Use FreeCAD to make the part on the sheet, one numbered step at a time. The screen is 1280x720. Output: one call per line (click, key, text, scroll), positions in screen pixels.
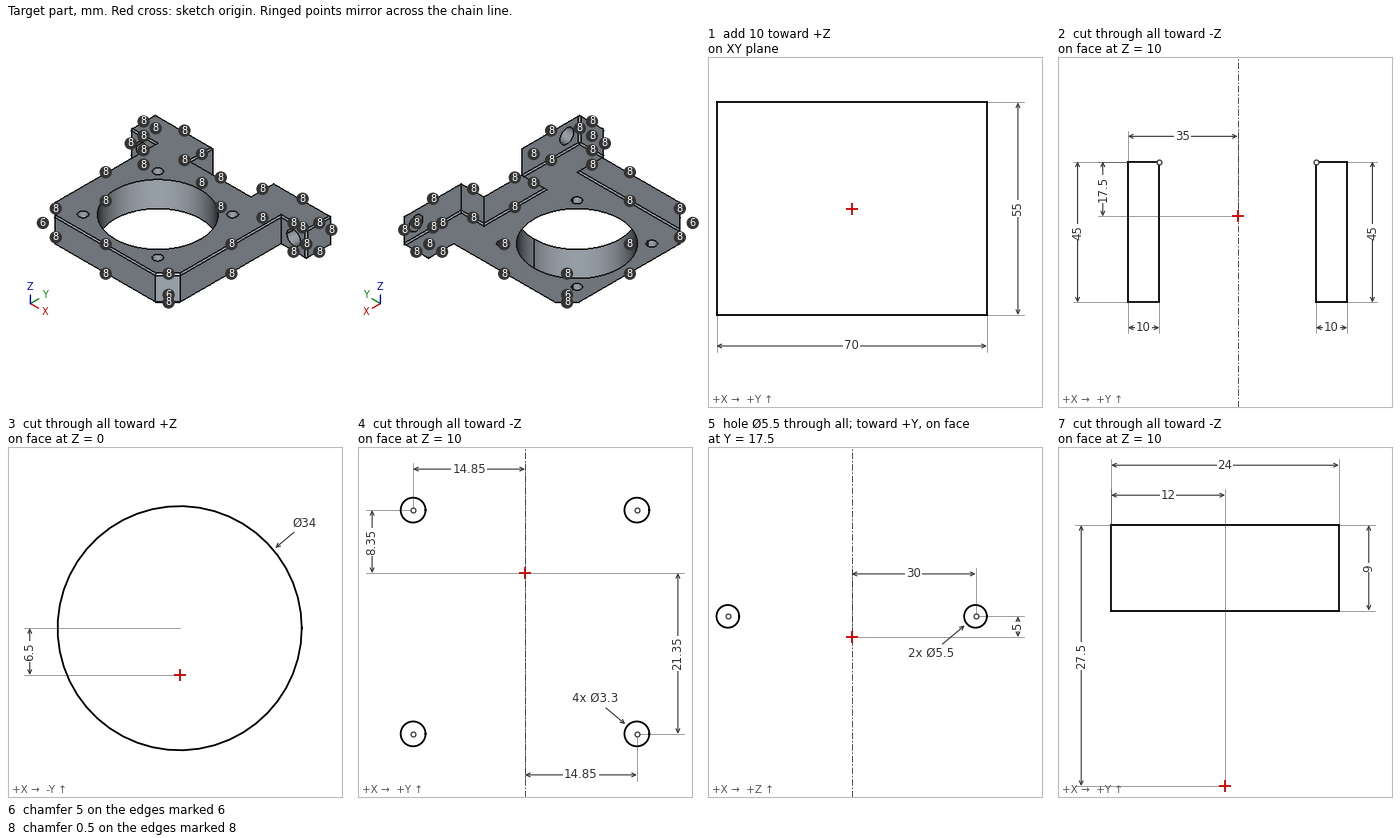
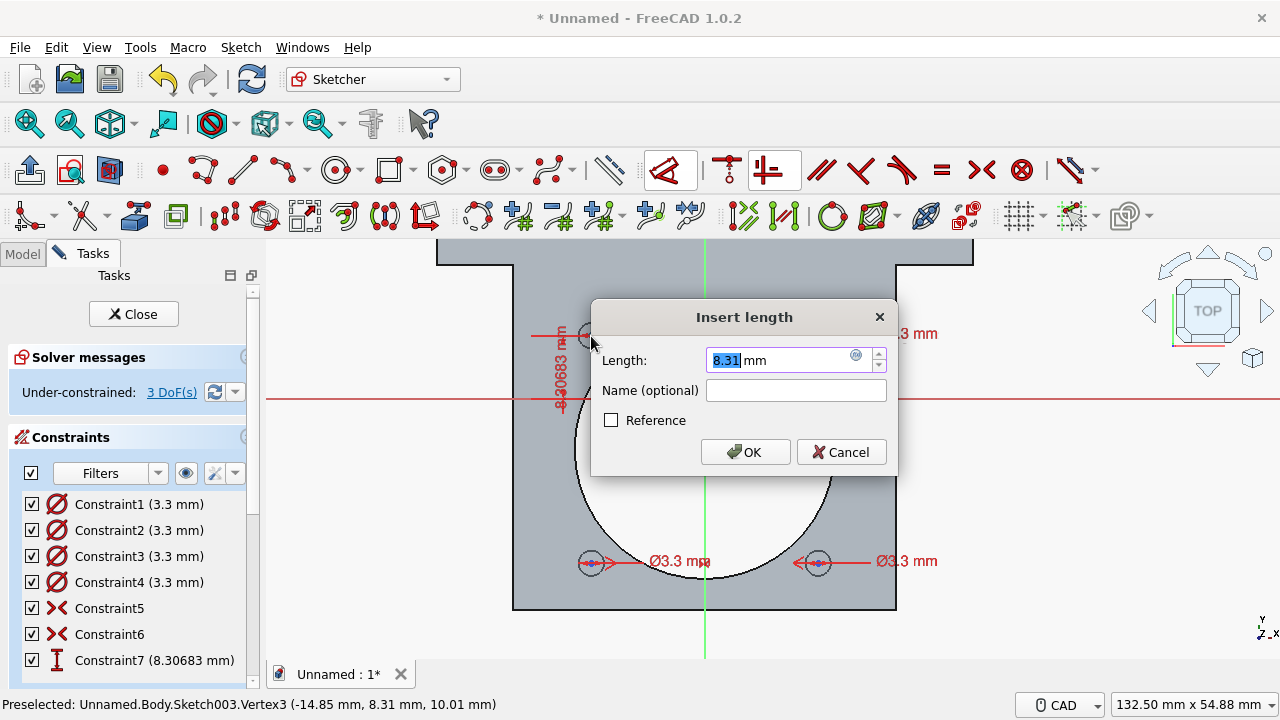
text(8.35)
key(Return)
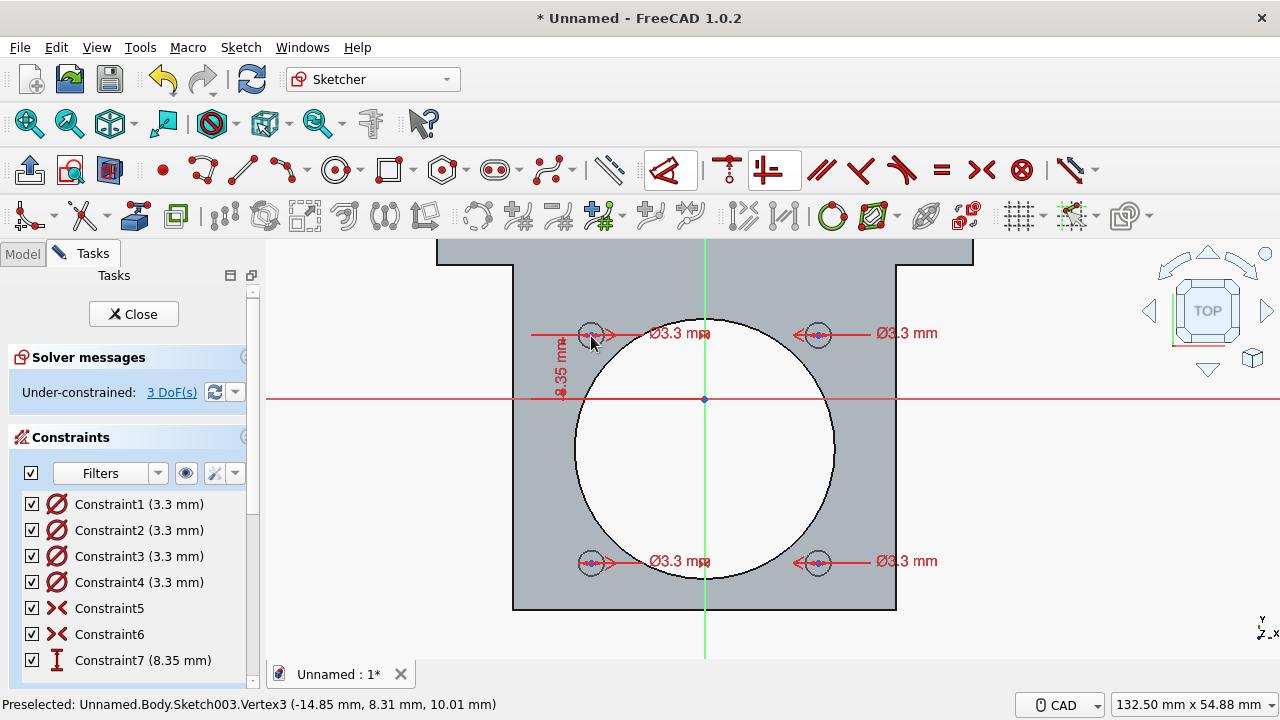
click(818, 563)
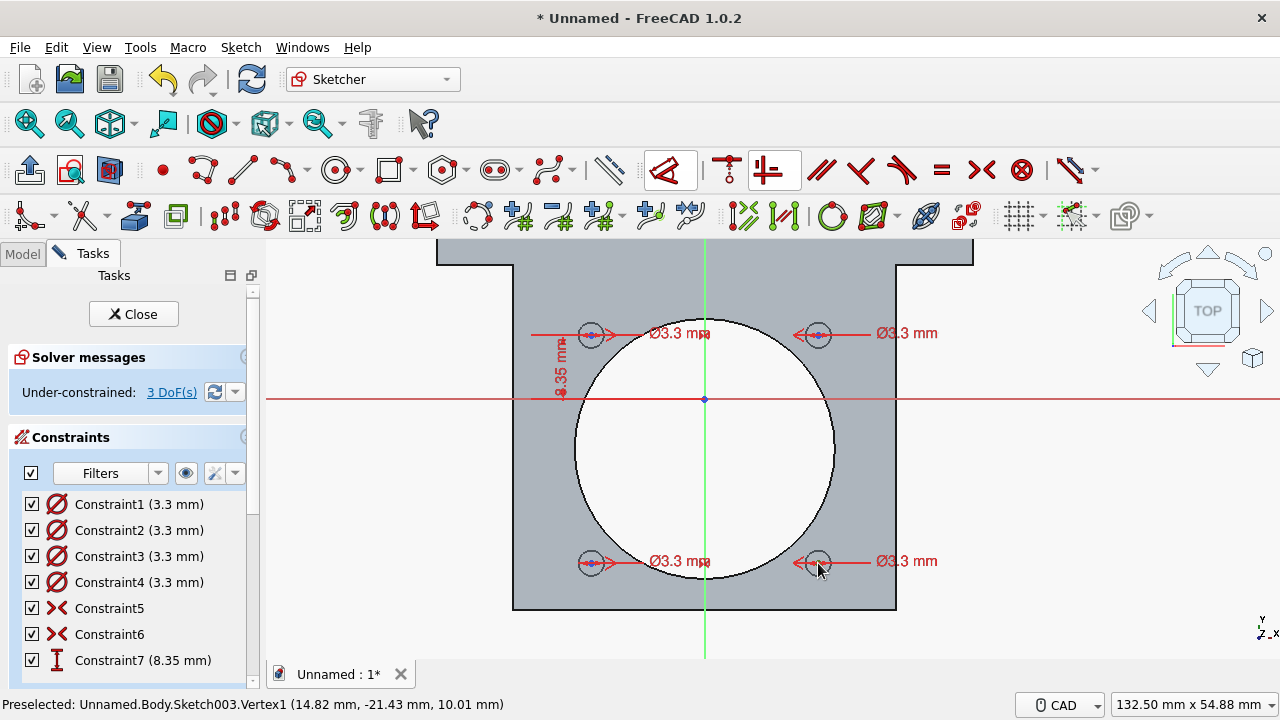
key(l)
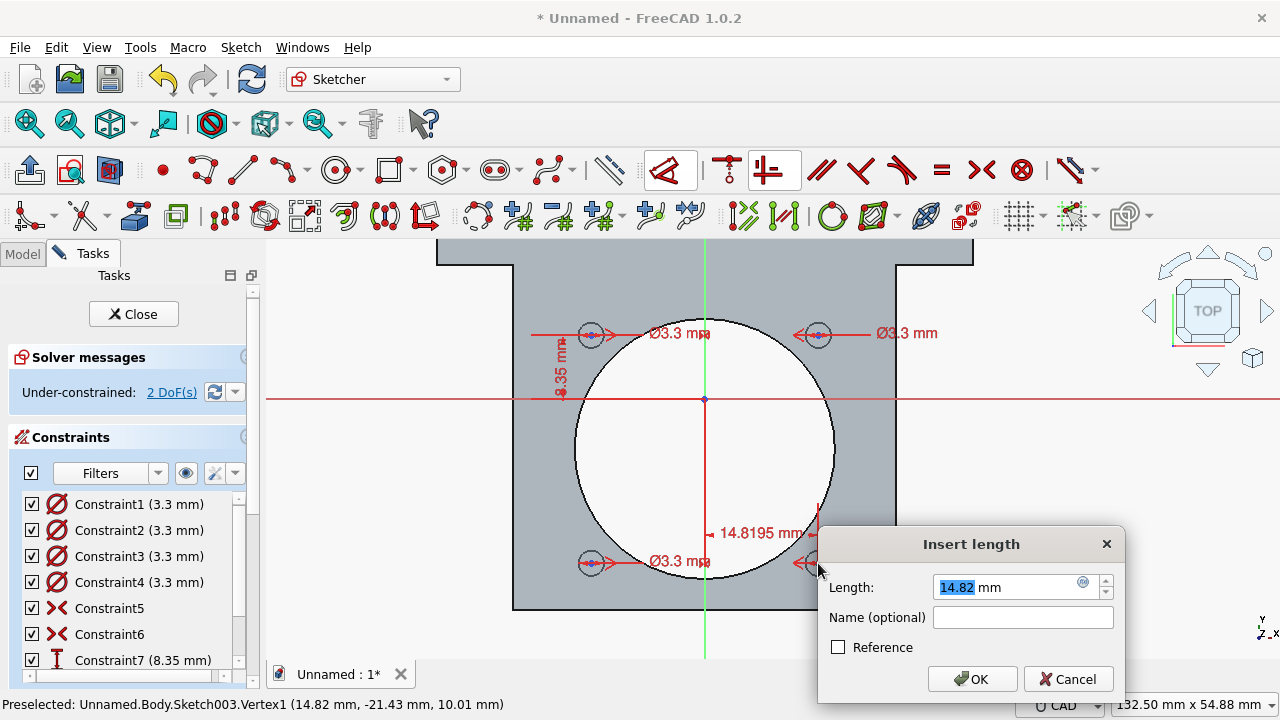
text(14.85)
key(Return)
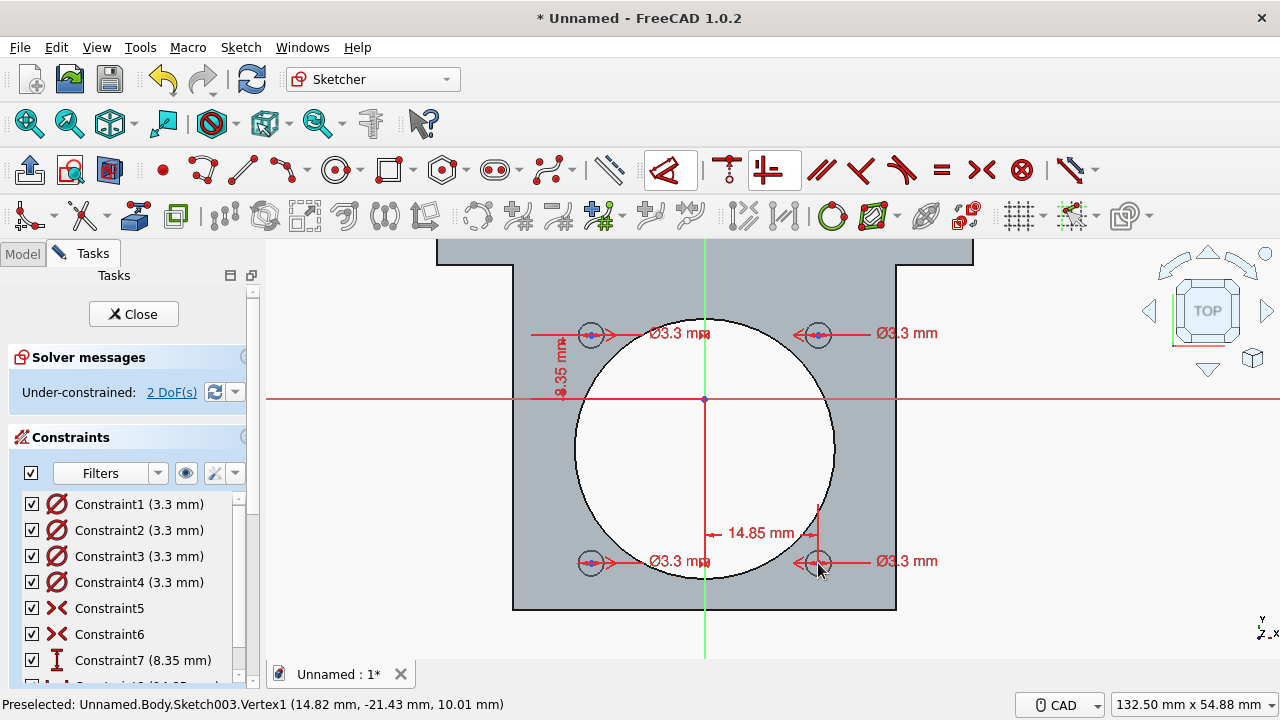
click(818, 563)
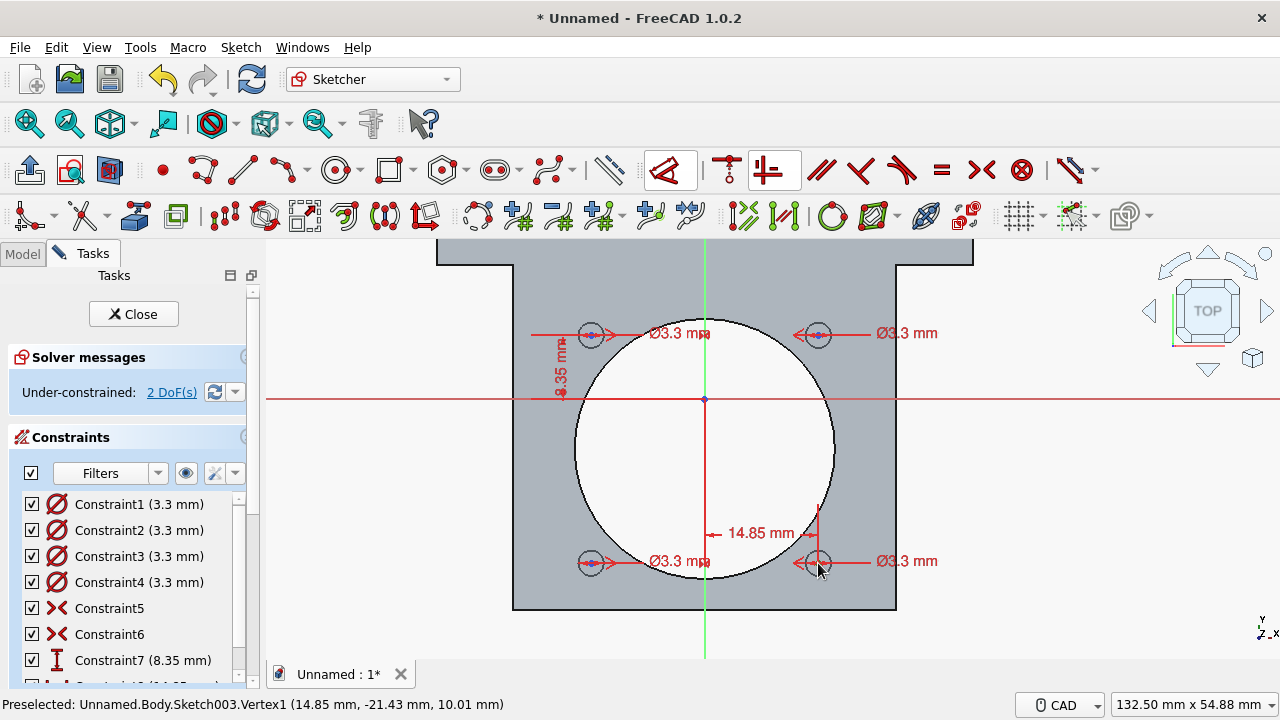
key(i)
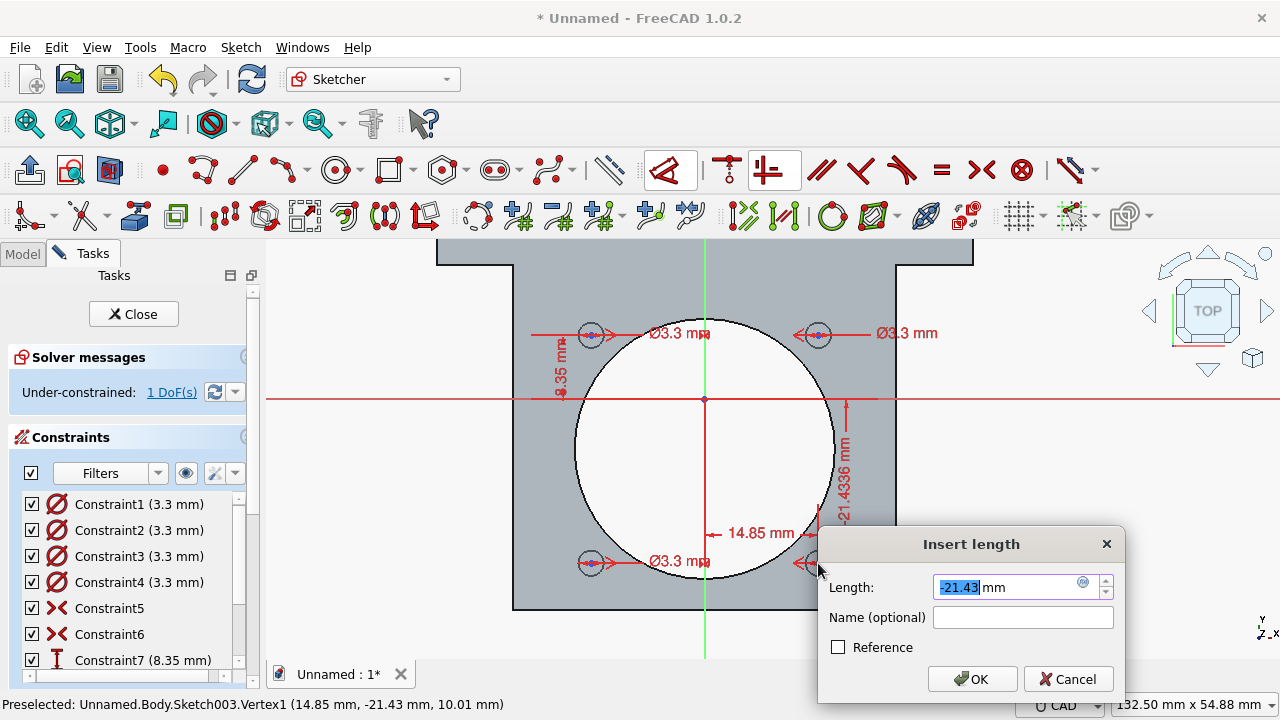
text(-21.35)
key(Return)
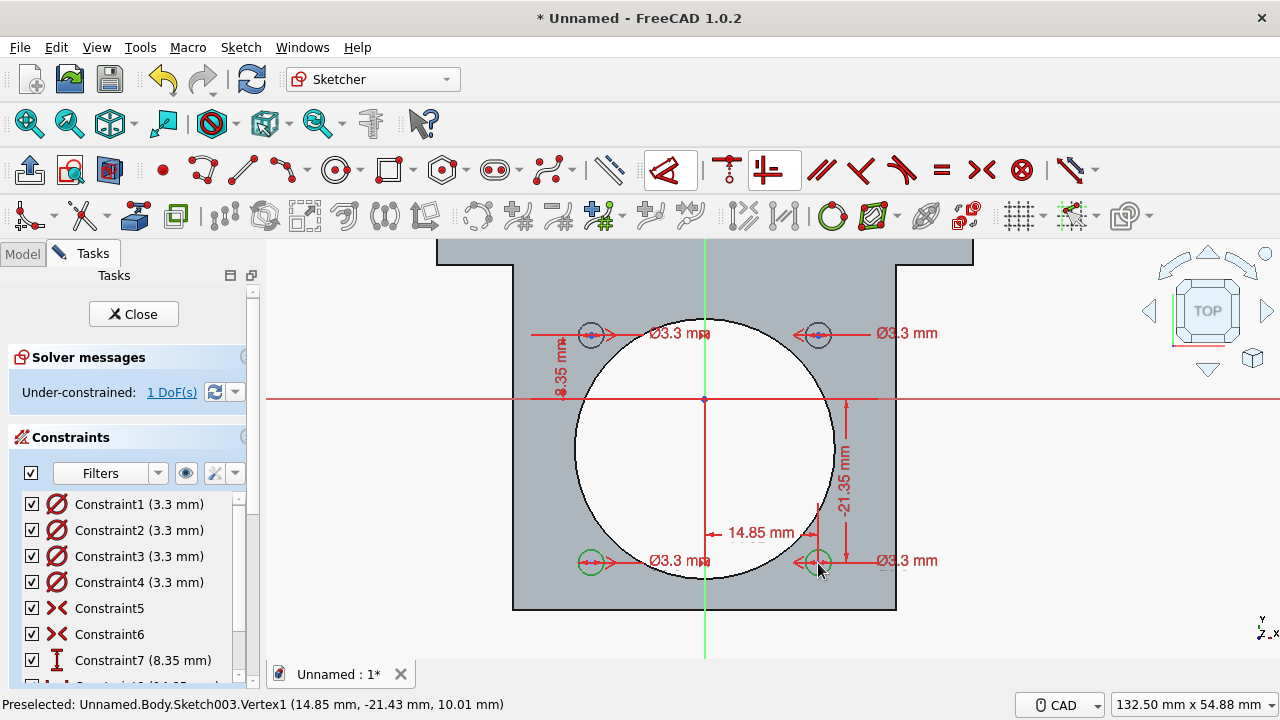
click(591, 335)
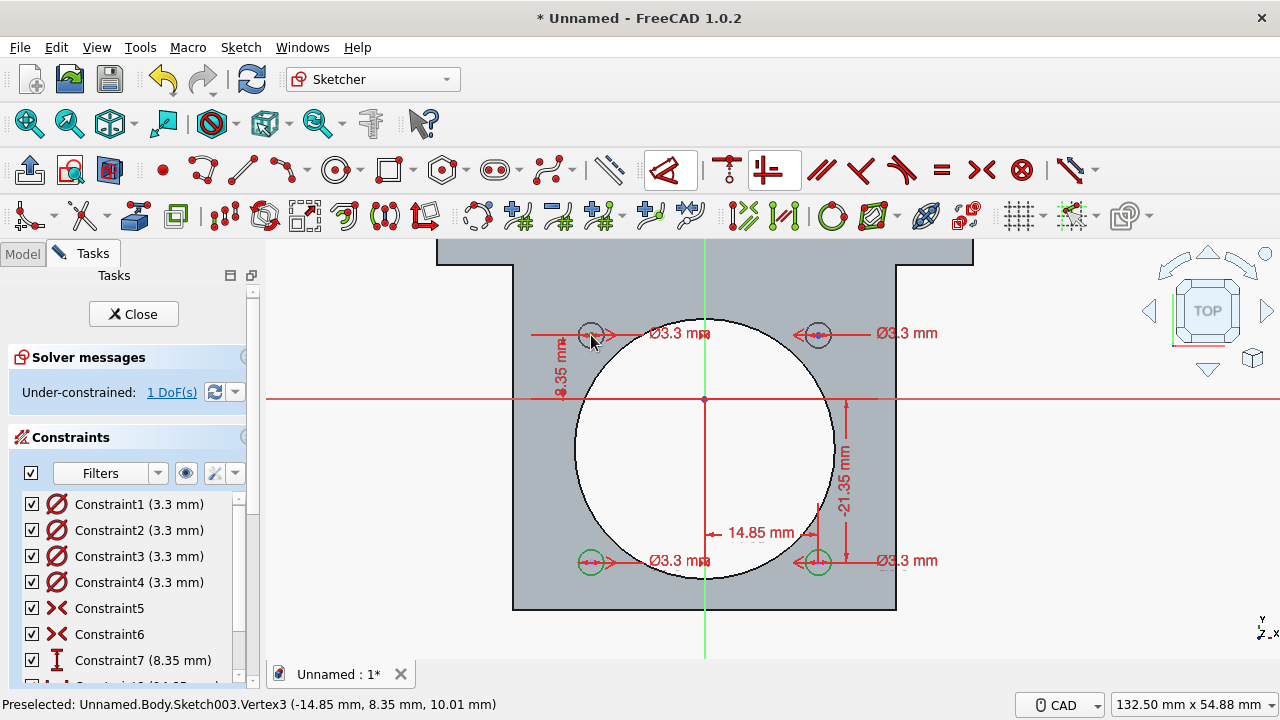
key(l)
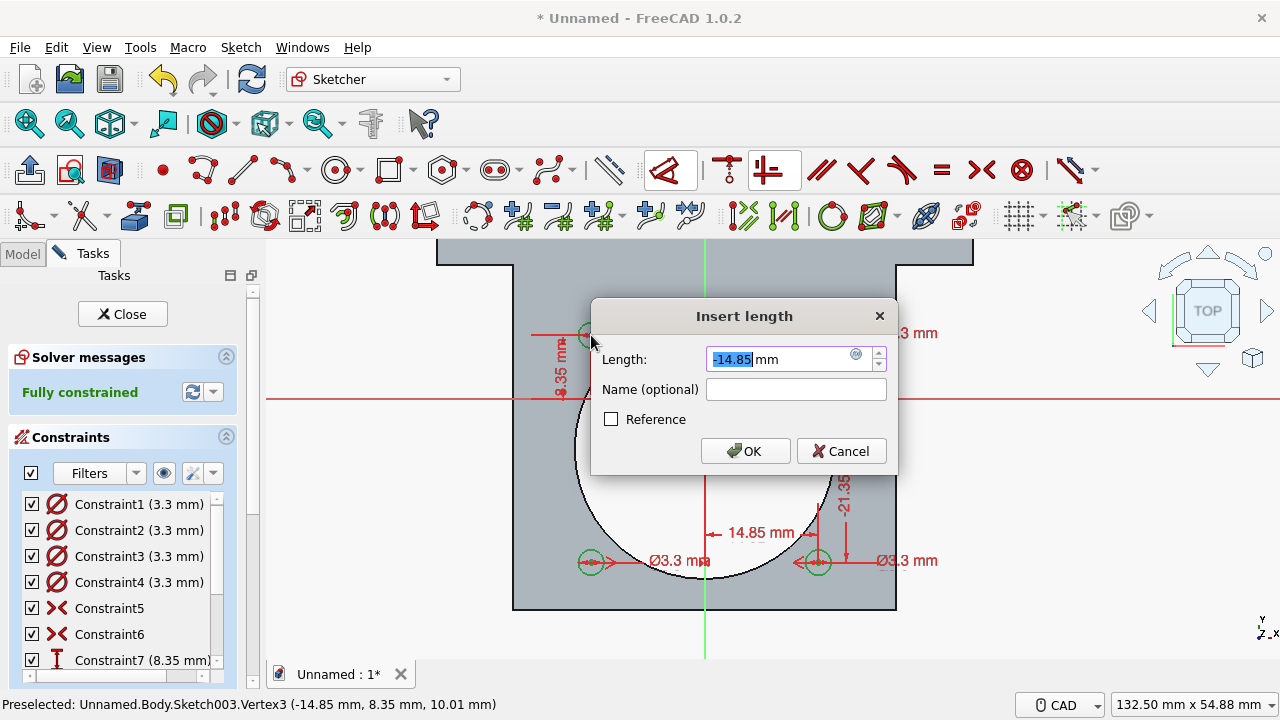
text(-14.85)
key(Return)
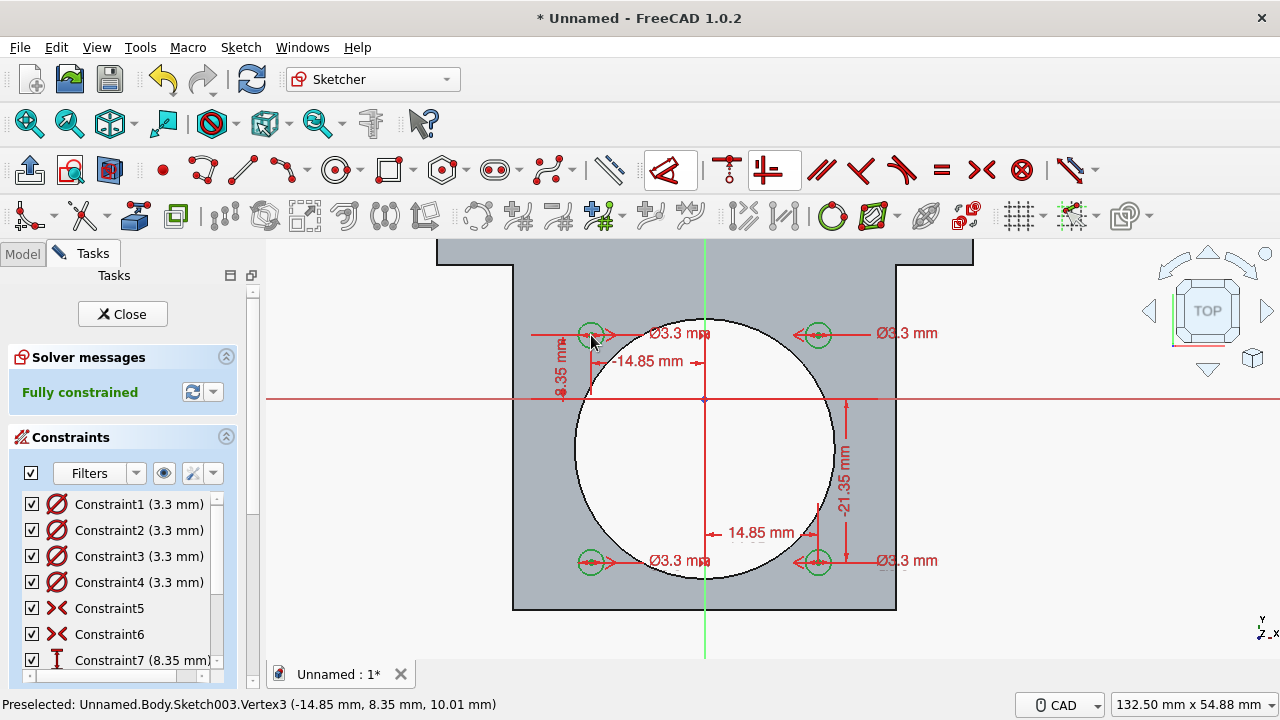
click(123, 314)